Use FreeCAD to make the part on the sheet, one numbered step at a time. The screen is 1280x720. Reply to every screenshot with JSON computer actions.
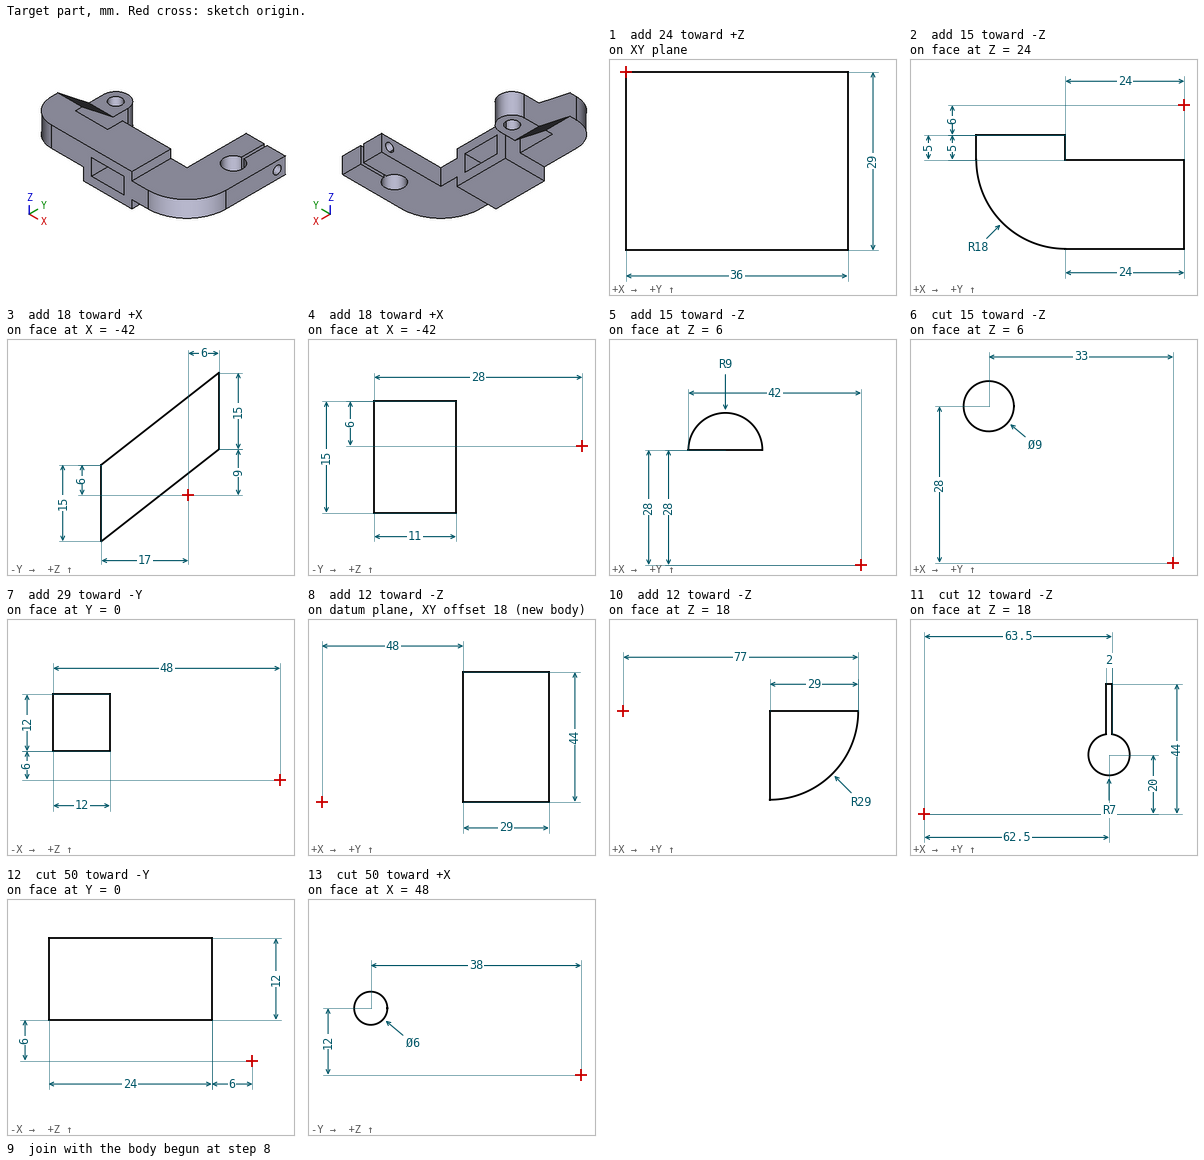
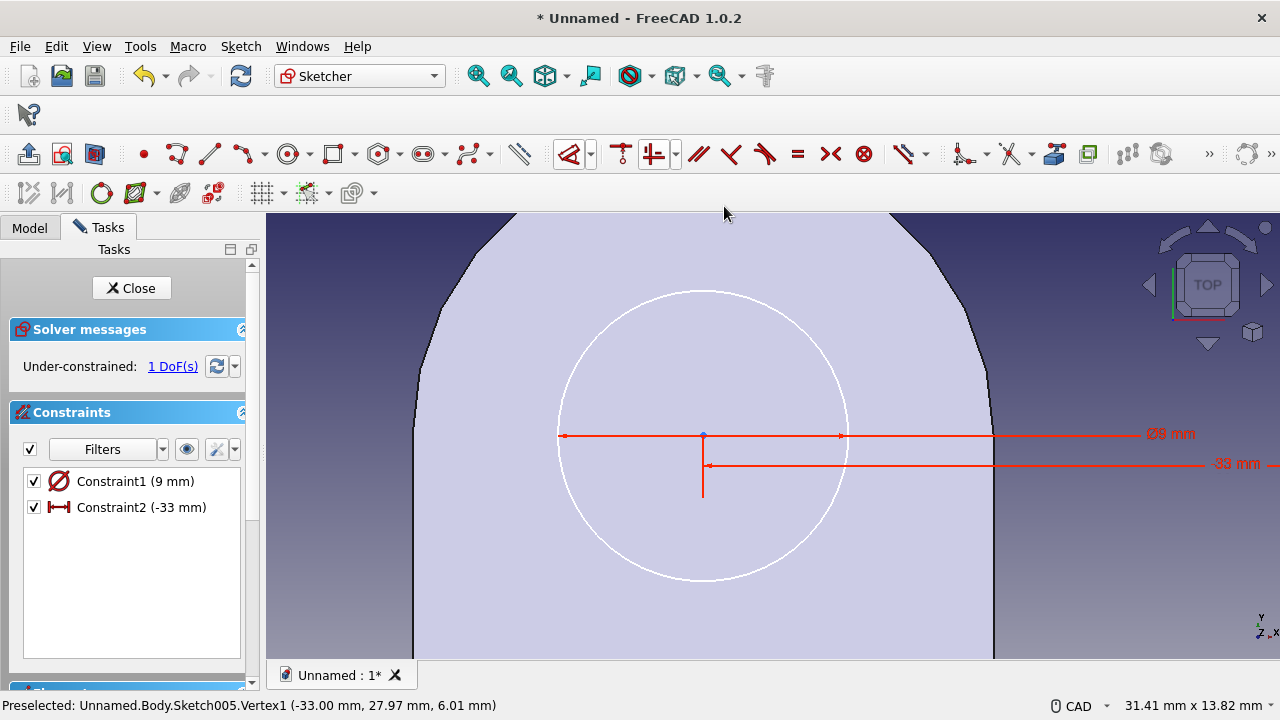
{"action": "left_click", "coordinate": [703, 436]}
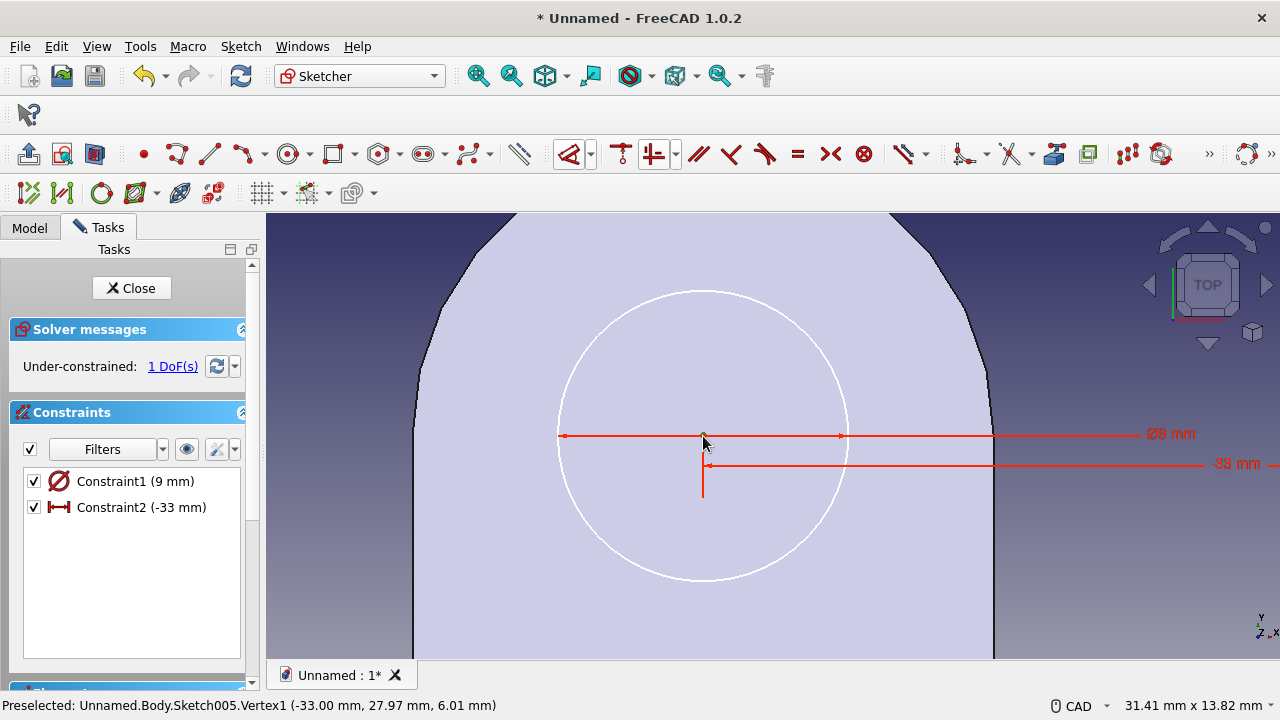
{"action": "key", "text": "i"}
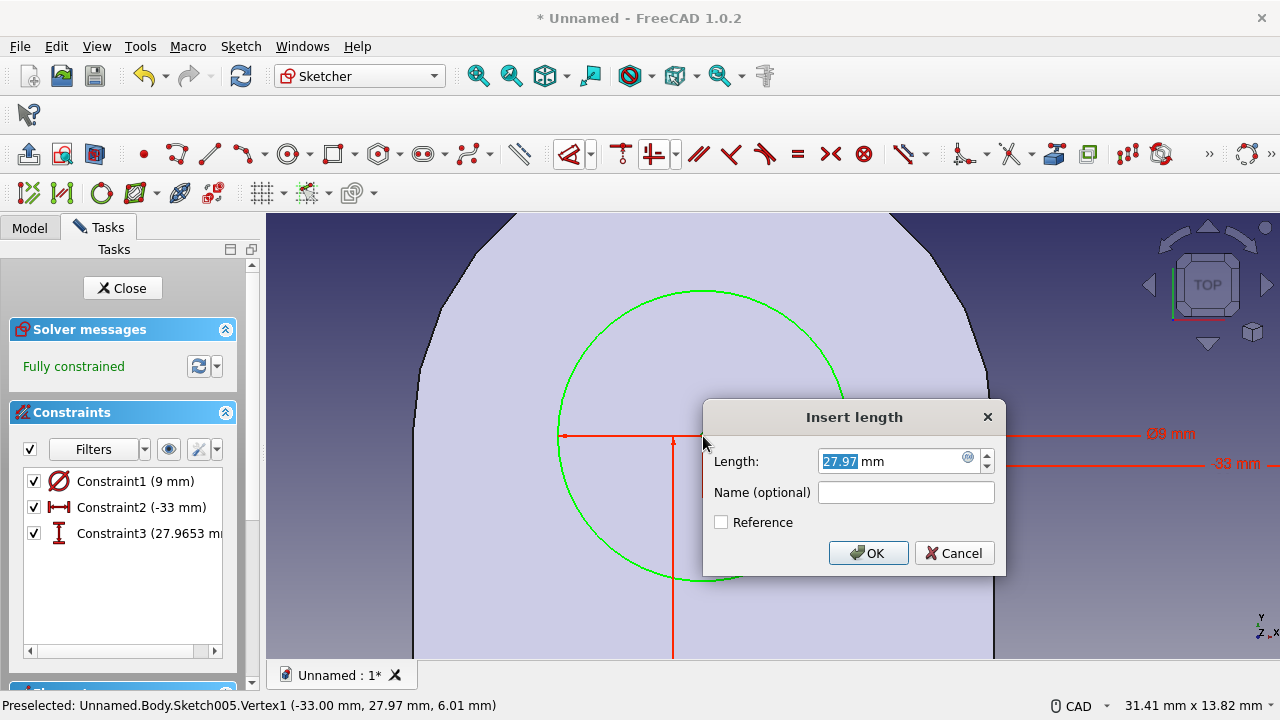
{"action": "type", "text": "28"}
{"action": "key", "text": "Return"}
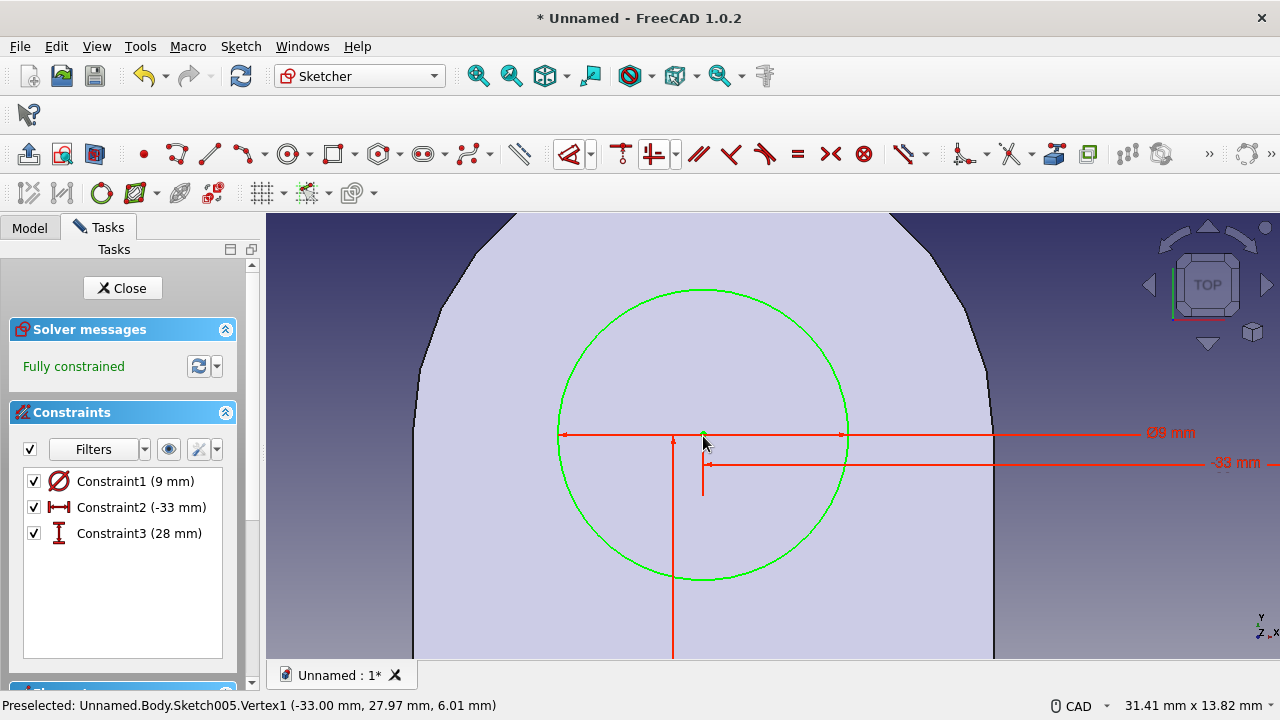
{"action": "left_click", "coordinate": [123, 288]}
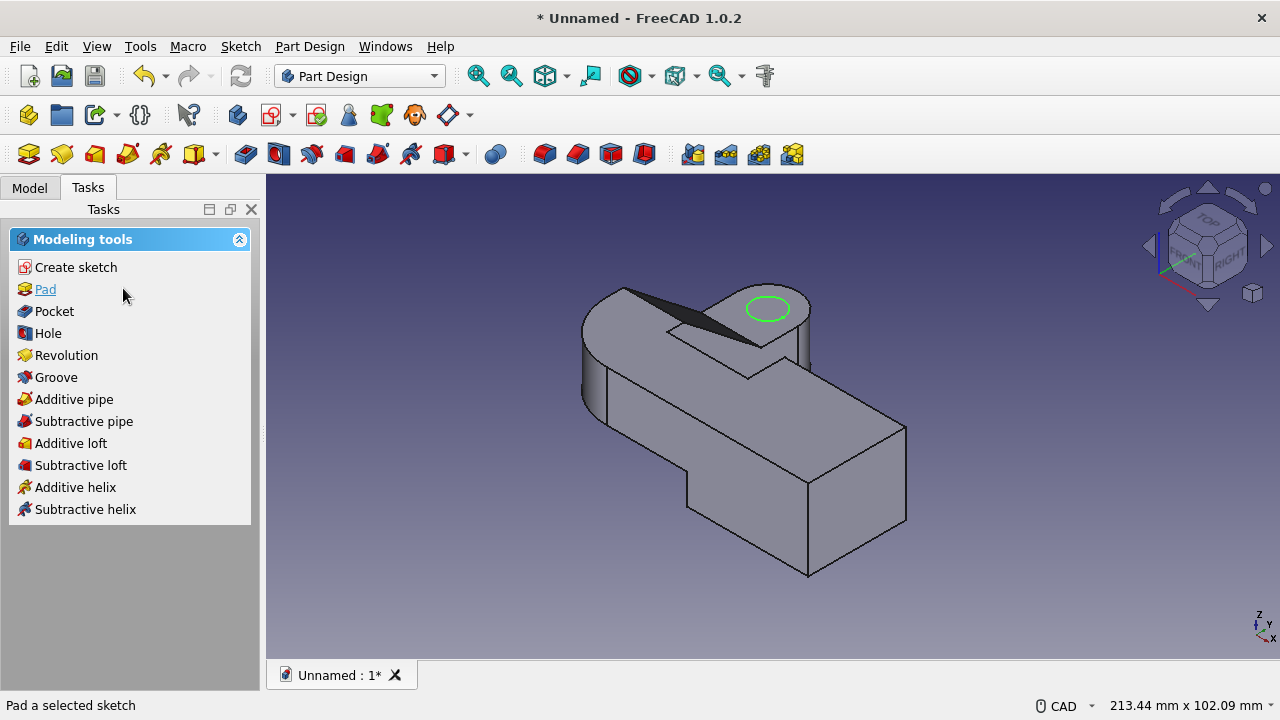
{"action": "left_click", "coordinate": [246, 154]}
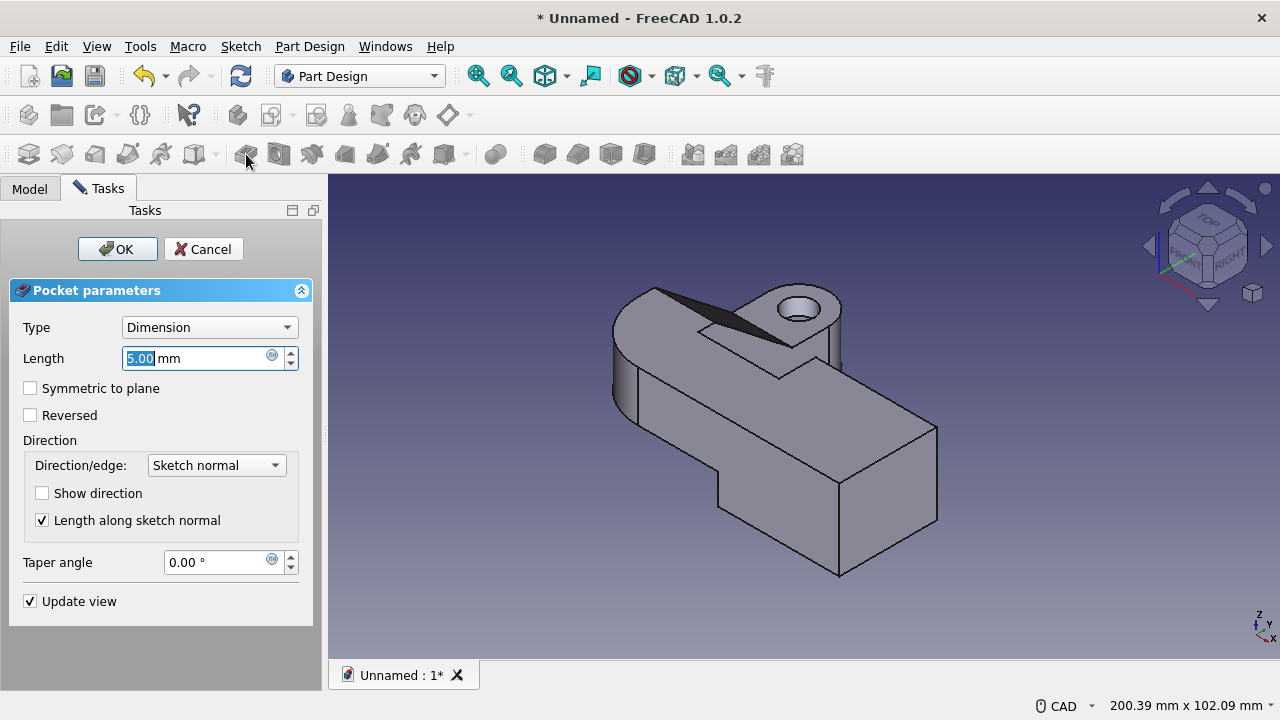
{"action": "type", "text": "15"}
{"action": "key", "text": "Tab"}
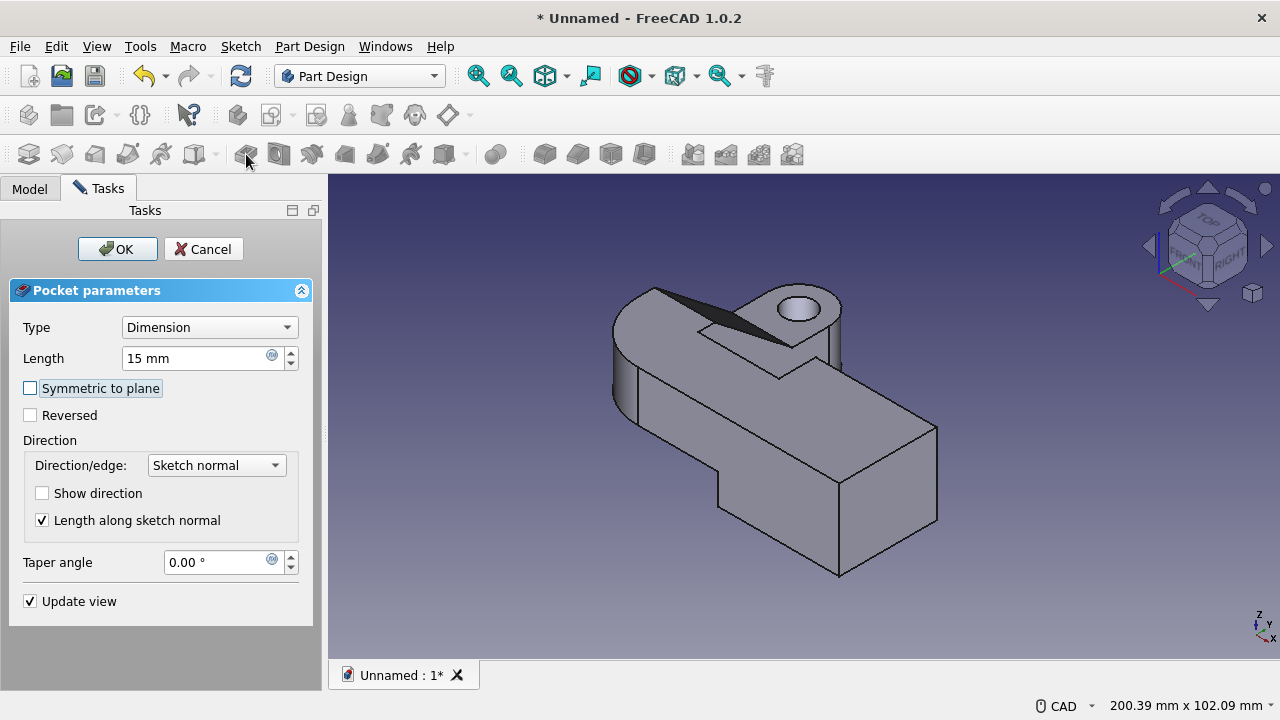
{"action": "left_click", "coordinate": [118, 249]}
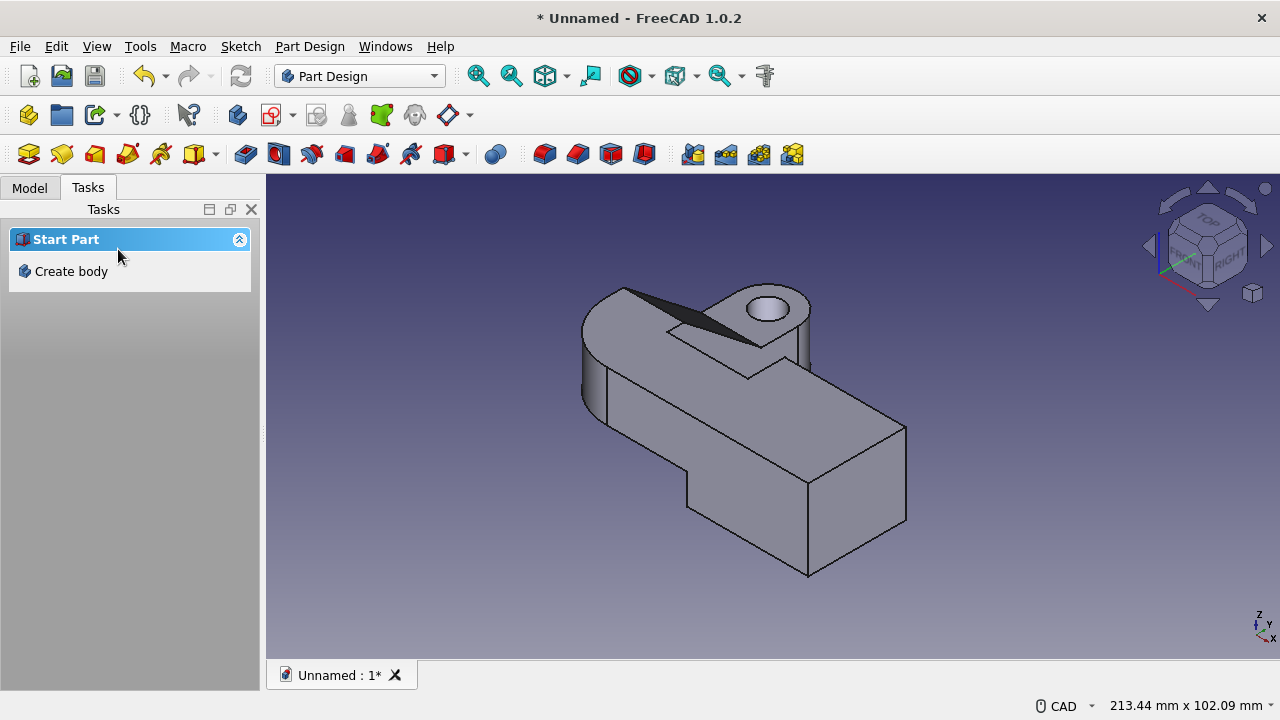
{"action": "key", "text": "4"}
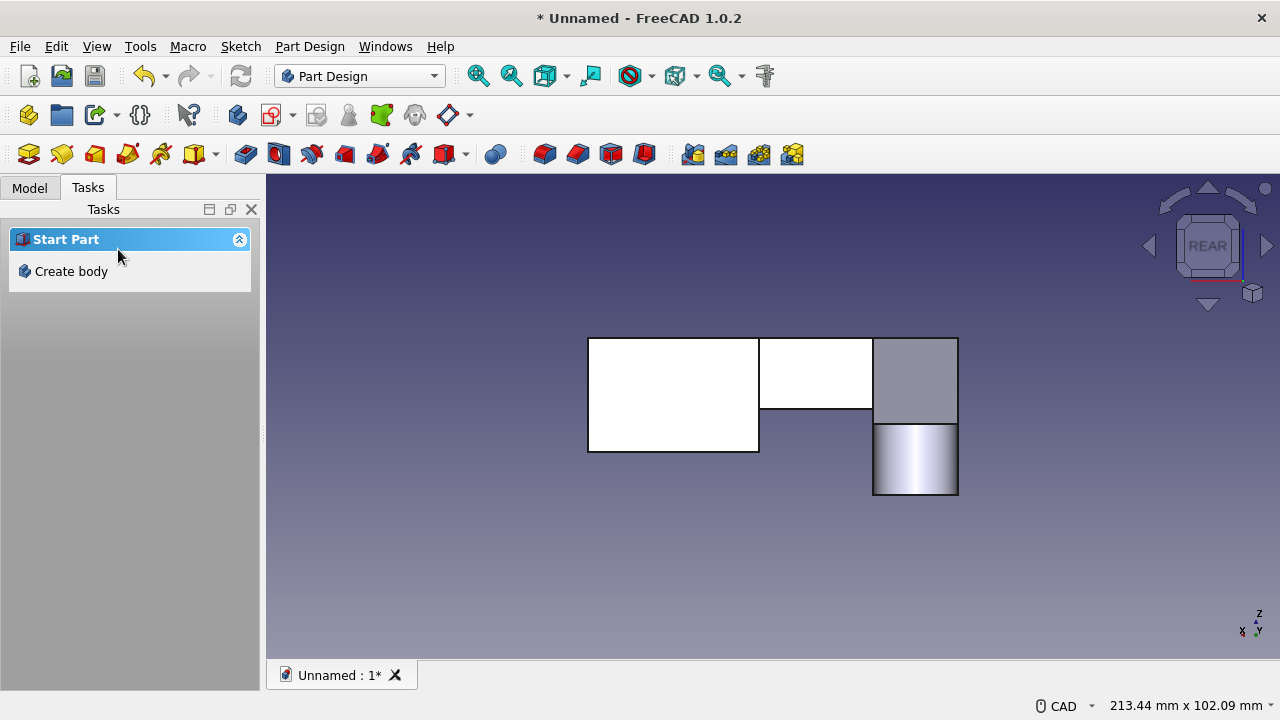
{"action": "left_click", "coordinate": [479, 76]}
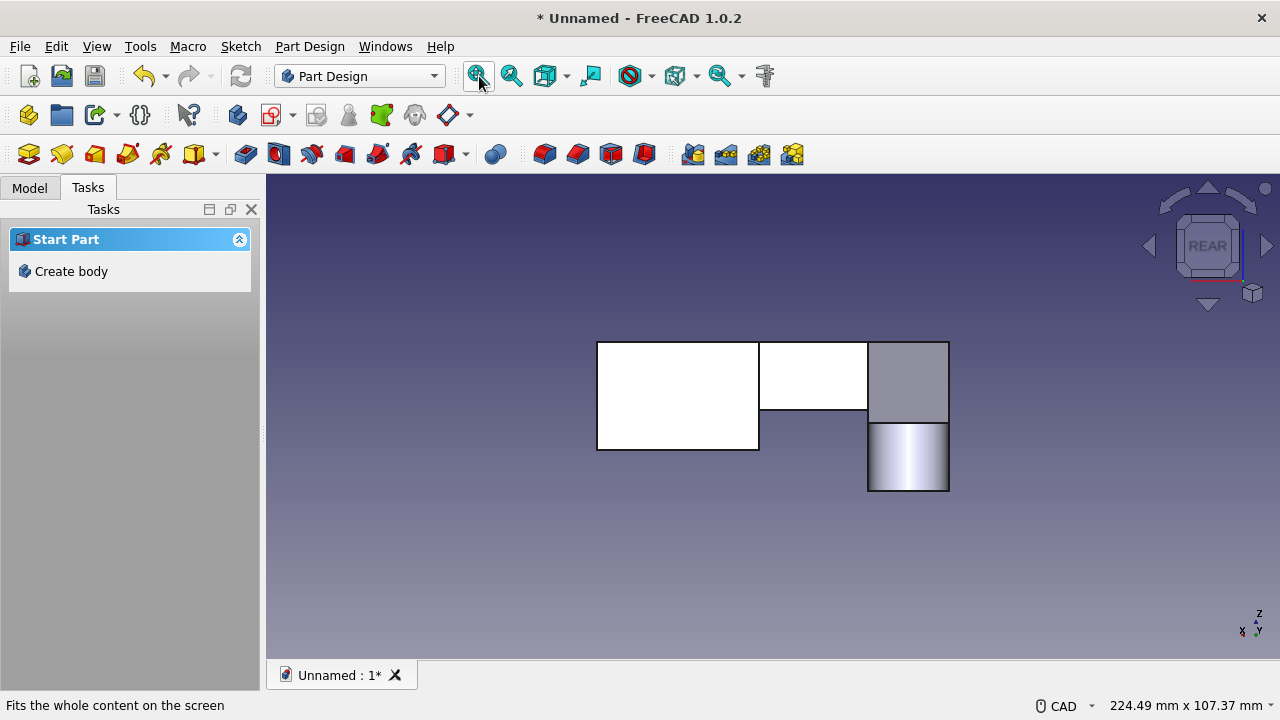
{"action": "left_click", "coordinate": [655, 395]}